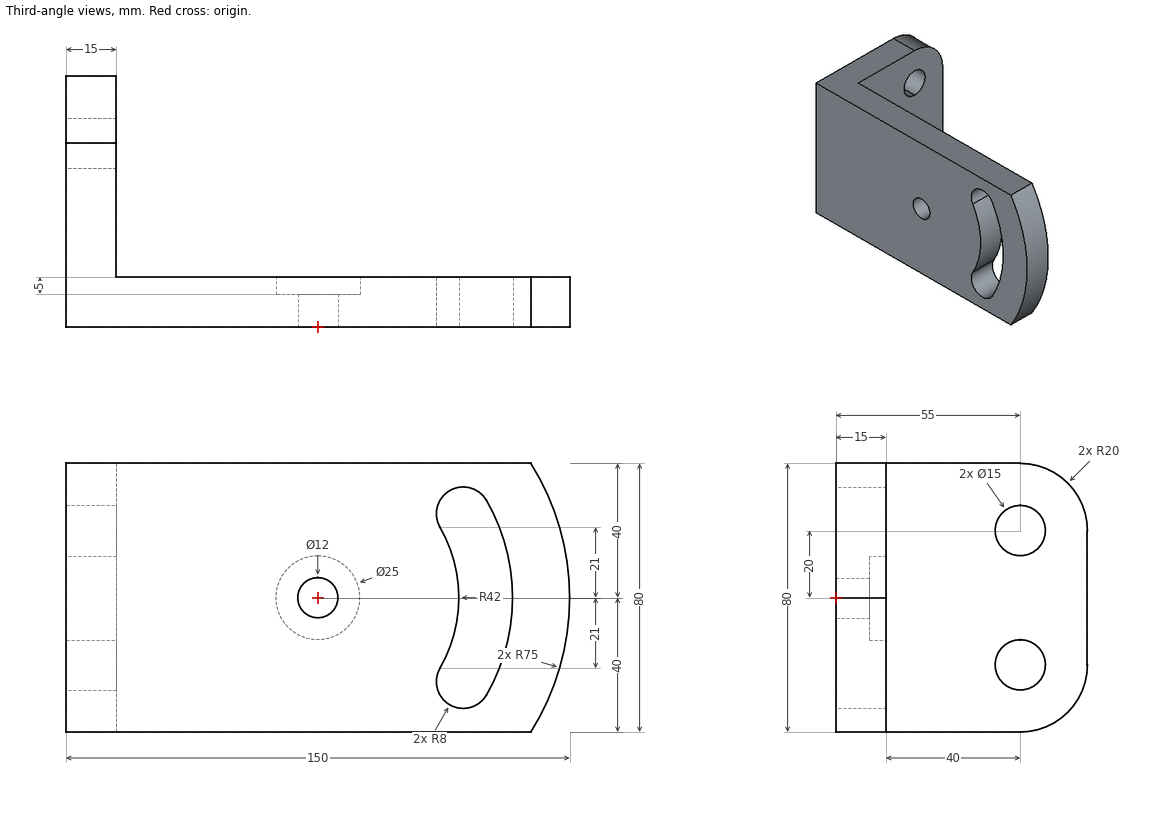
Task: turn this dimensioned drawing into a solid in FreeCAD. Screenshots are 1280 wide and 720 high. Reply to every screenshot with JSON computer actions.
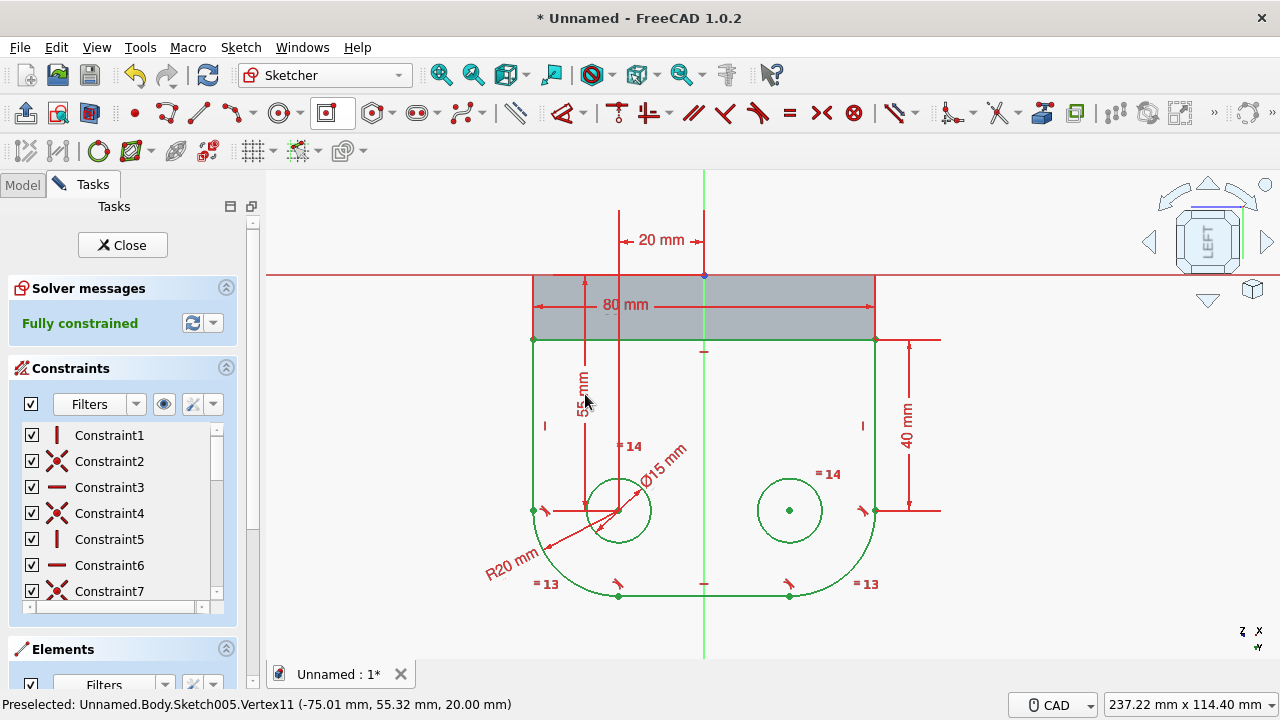
{"action": "left_click", "coordinate": [123, 245]}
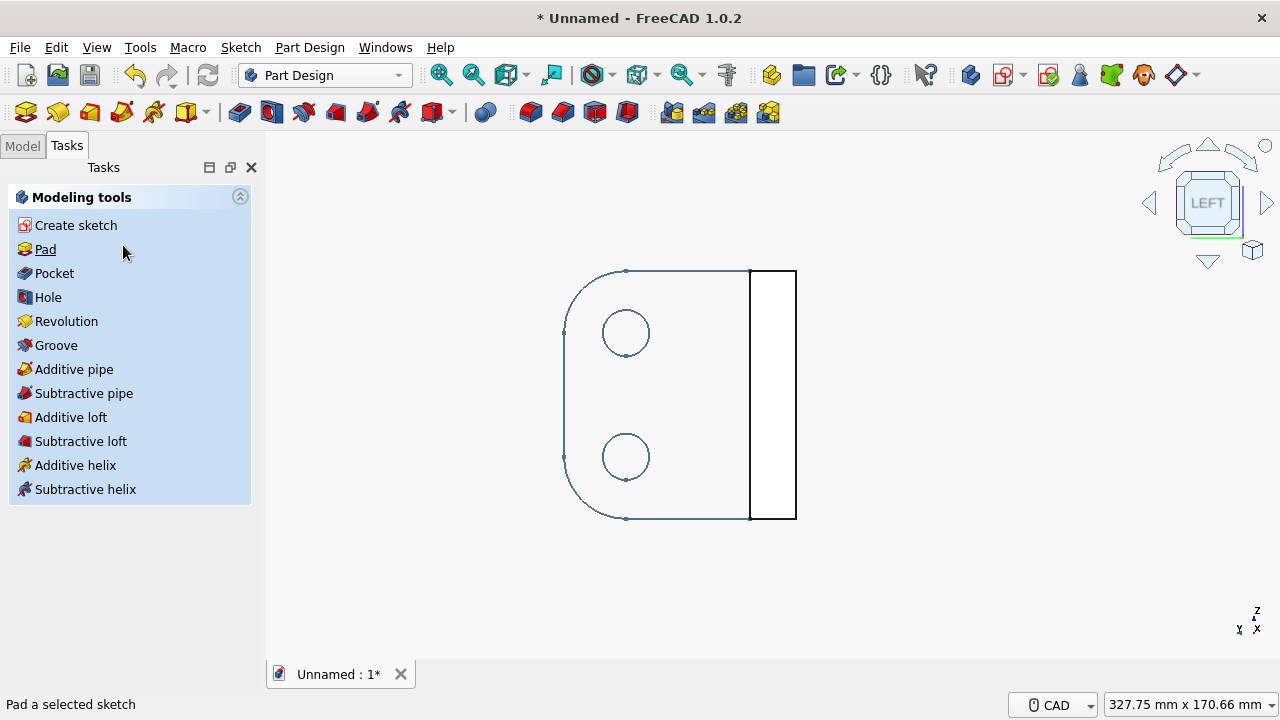
{"action": "left_click", "coordinate": [26, 112]}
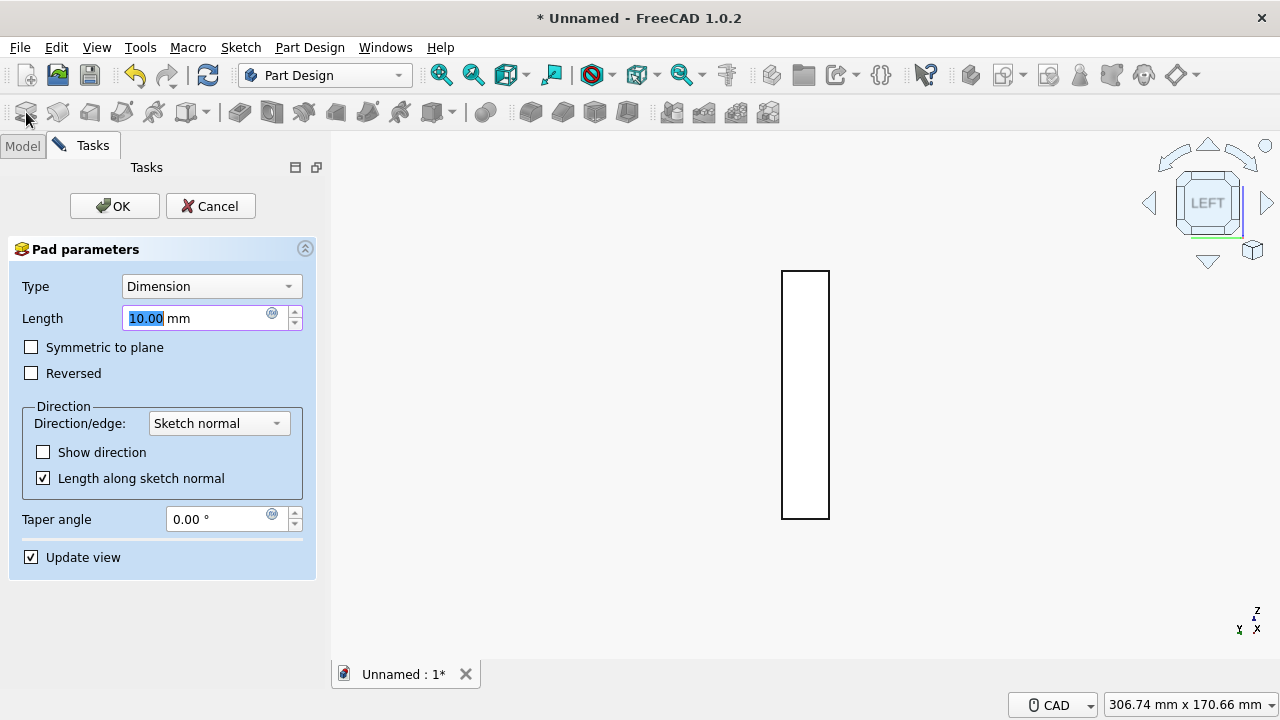
{"action": "type", "text": "15"}
{"action": "key", "text": "Tab"}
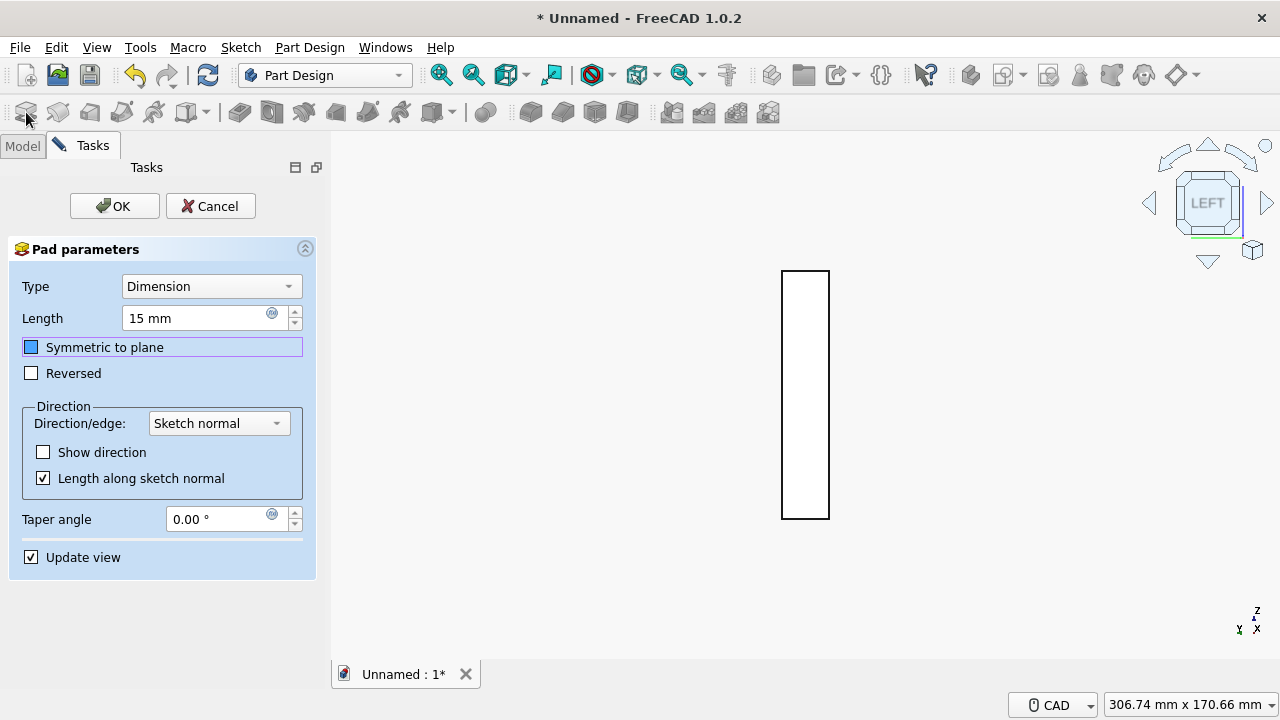
{"action": "left_click", "coordinate": [30, 373]}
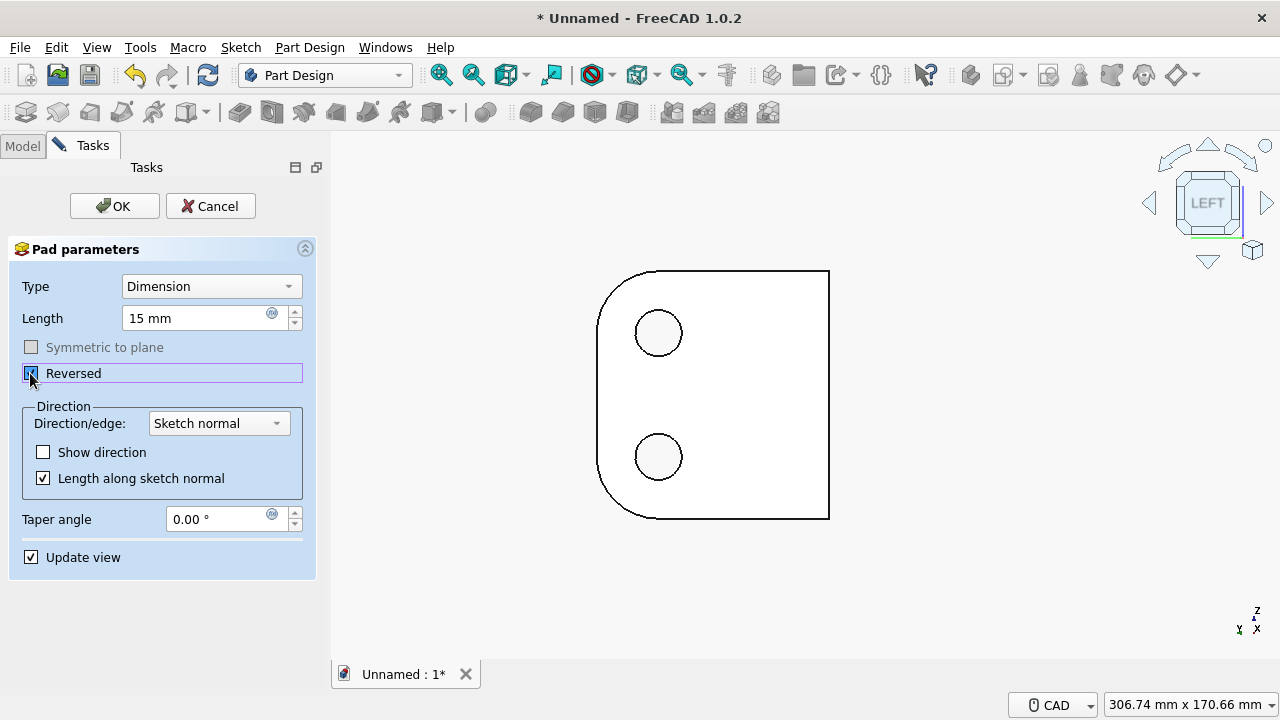
{"action": "left_click", "coordinate": [115, 206]}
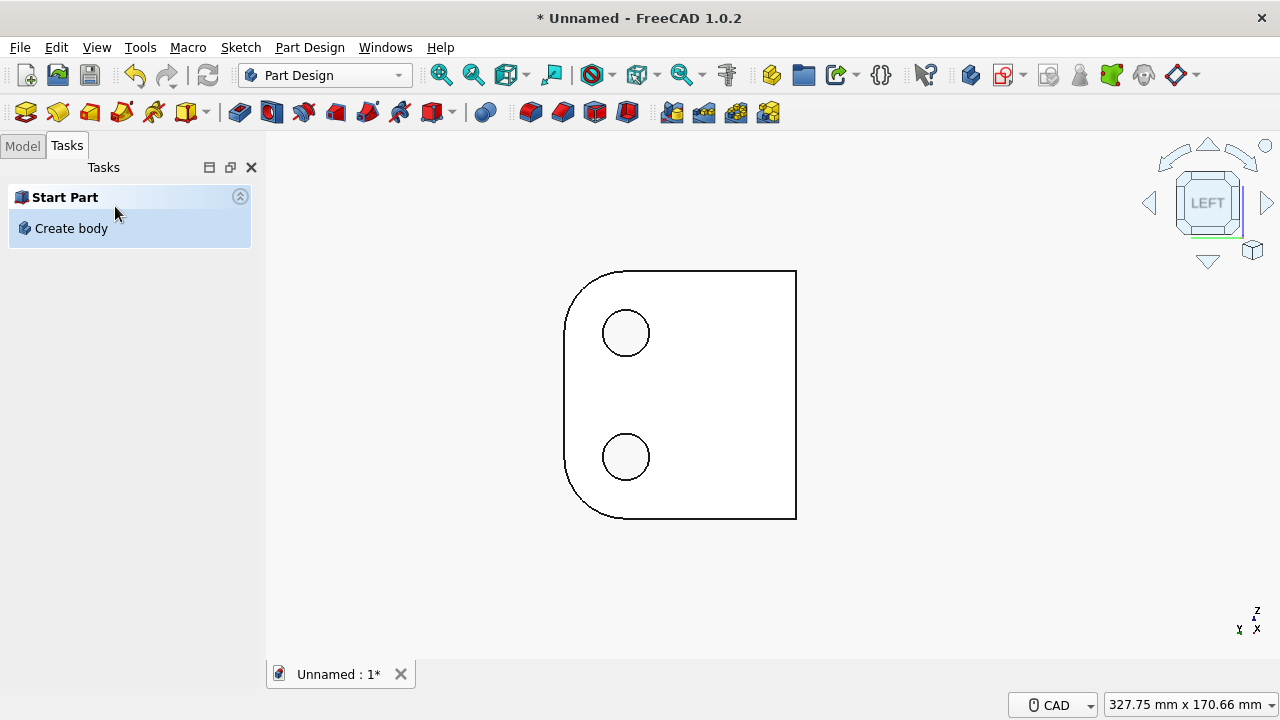
{"action": "key", "text": "0"}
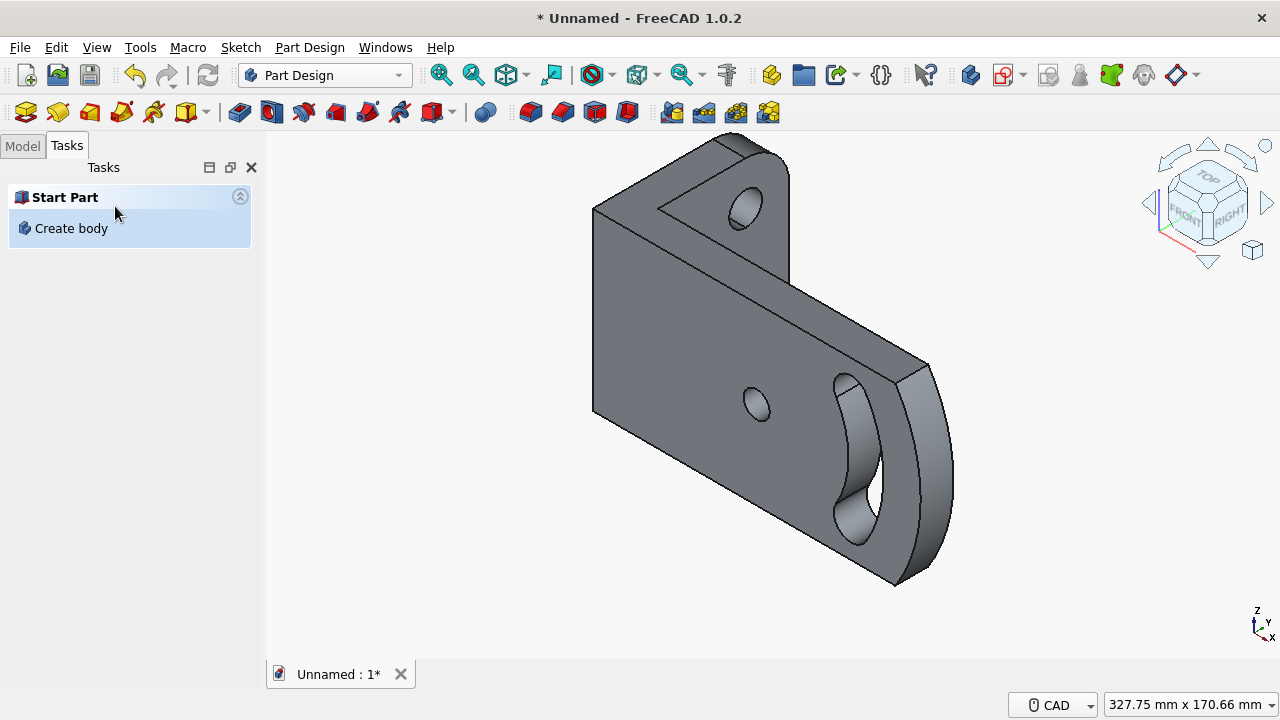
{"action": "left_click", "coordinate": [442, 76]}